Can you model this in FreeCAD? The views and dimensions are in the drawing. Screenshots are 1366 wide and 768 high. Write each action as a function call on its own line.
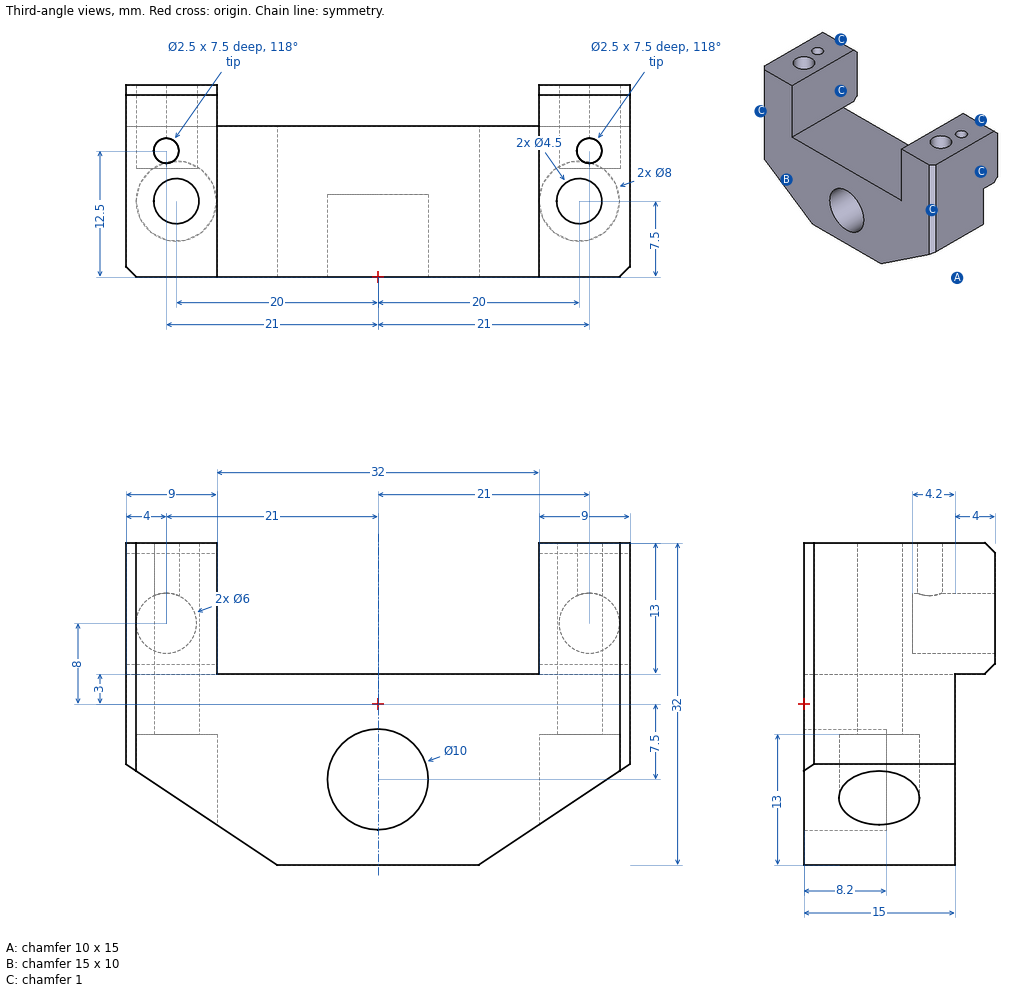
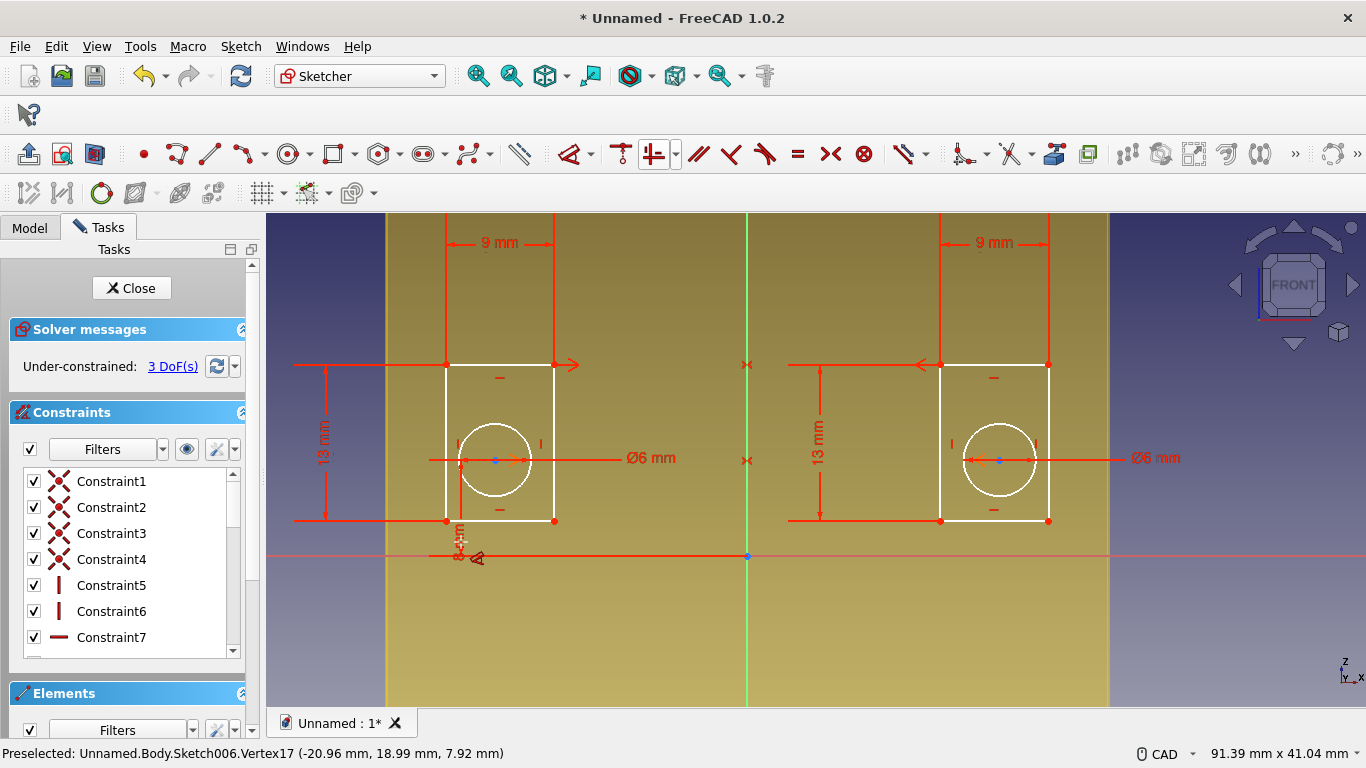
click(446, 521)
click(781, 539)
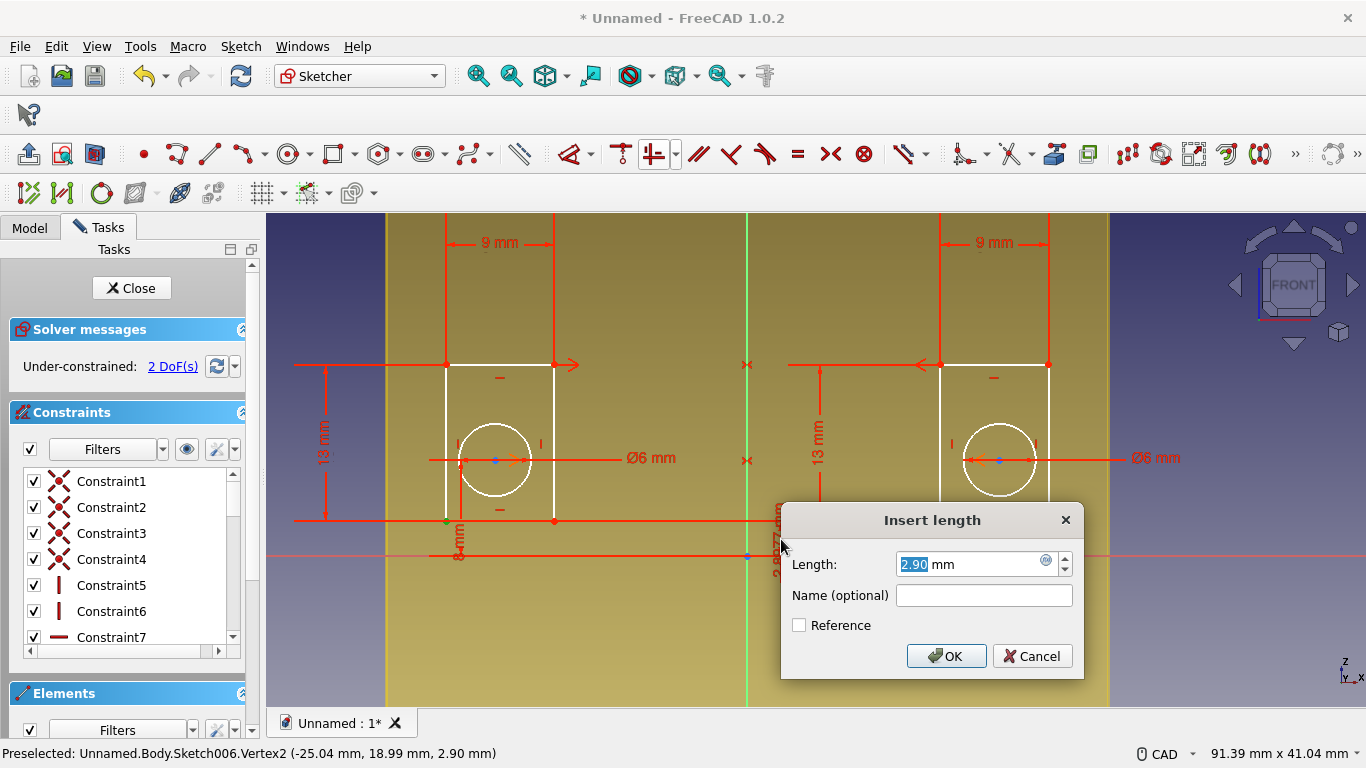
text(3)
key(Return)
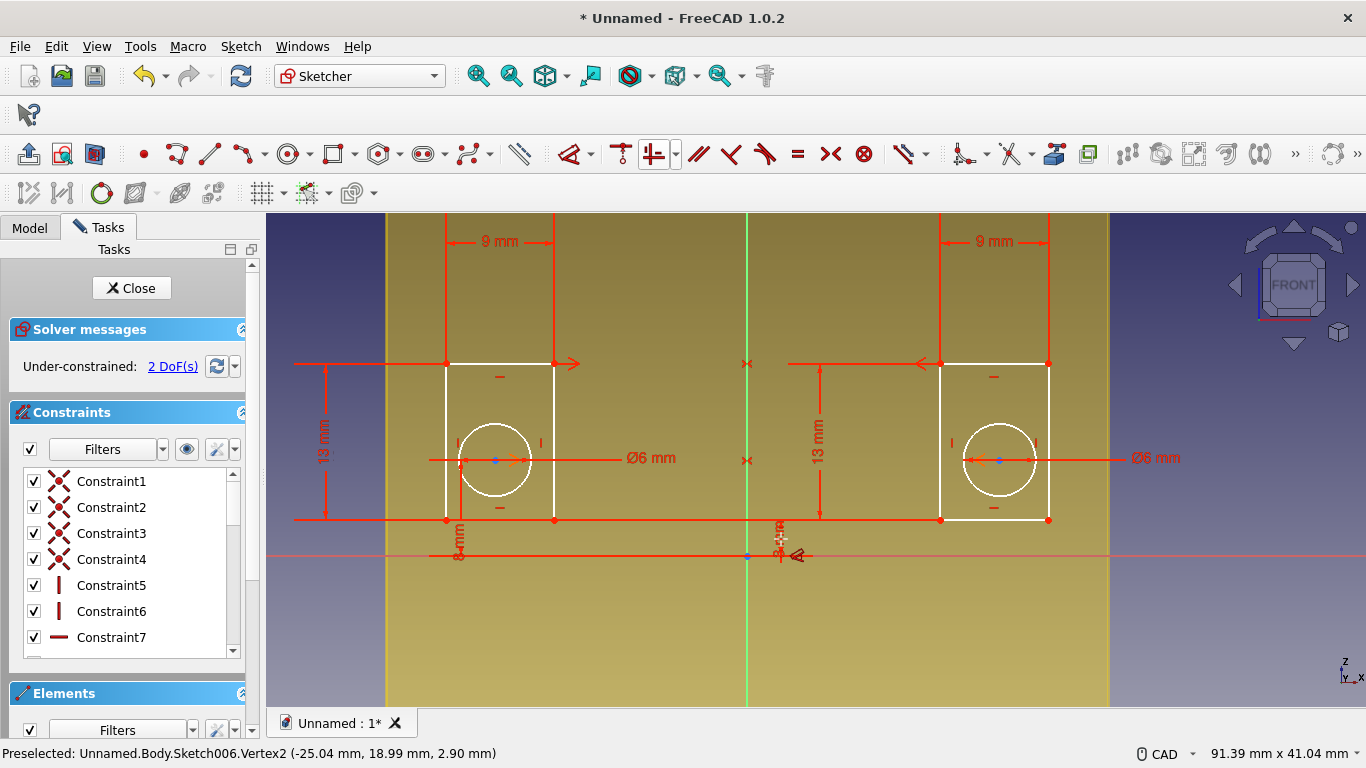
click(495, 460)
click(621, 590)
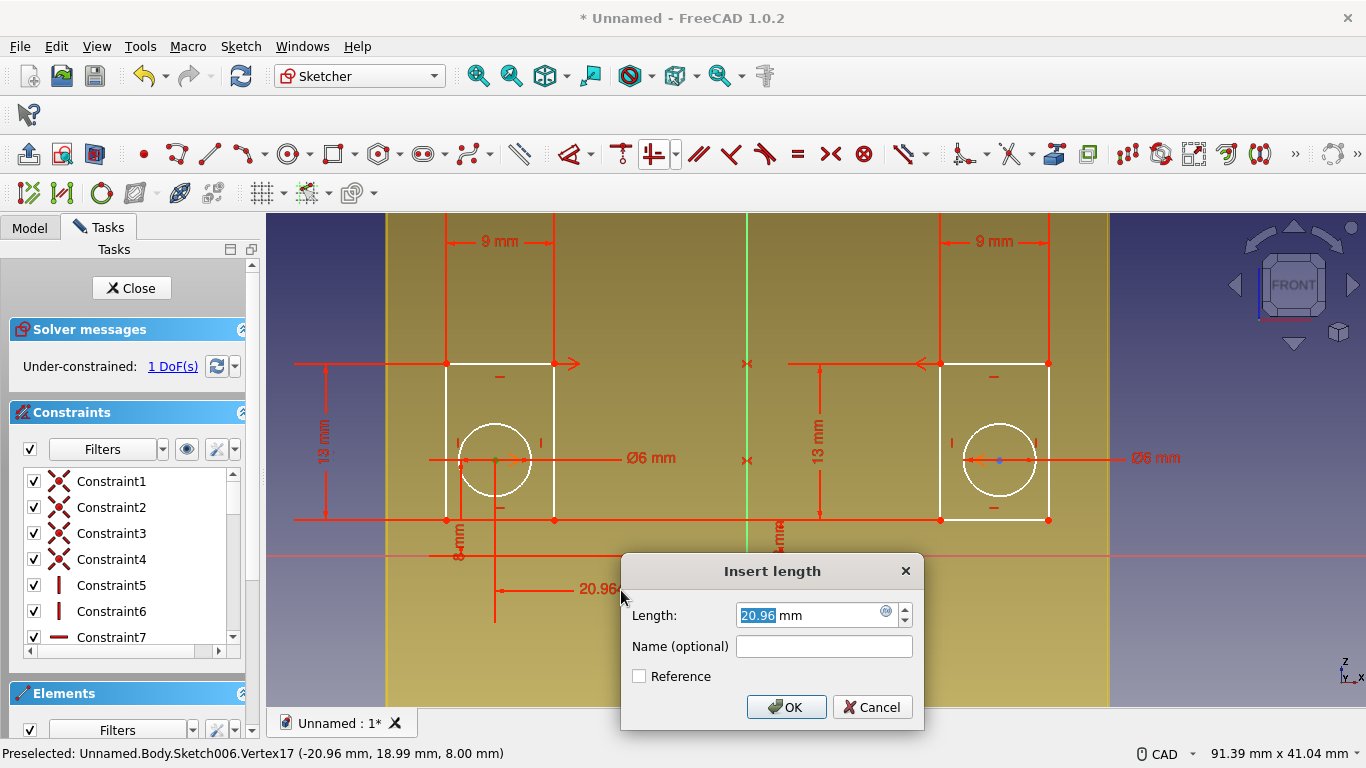
text(21)
key(Return)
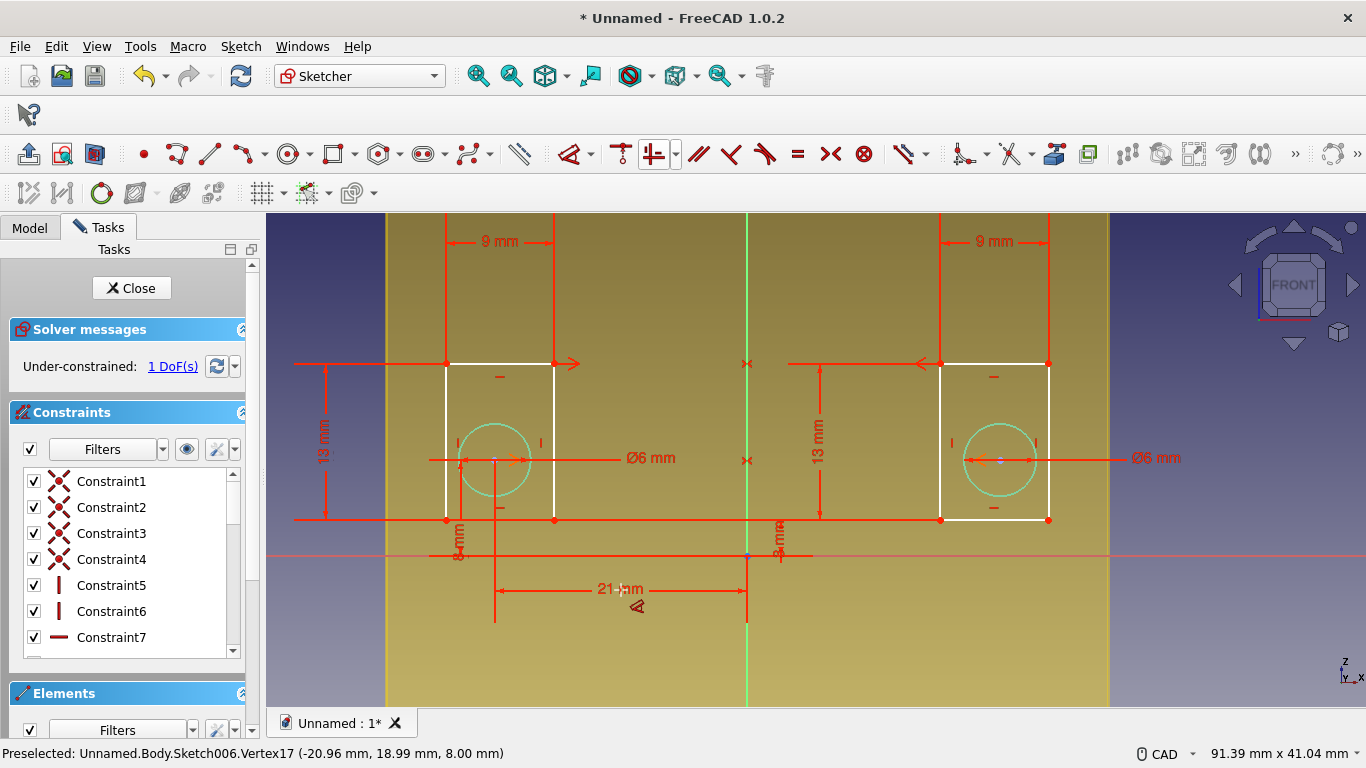
click(446, 520)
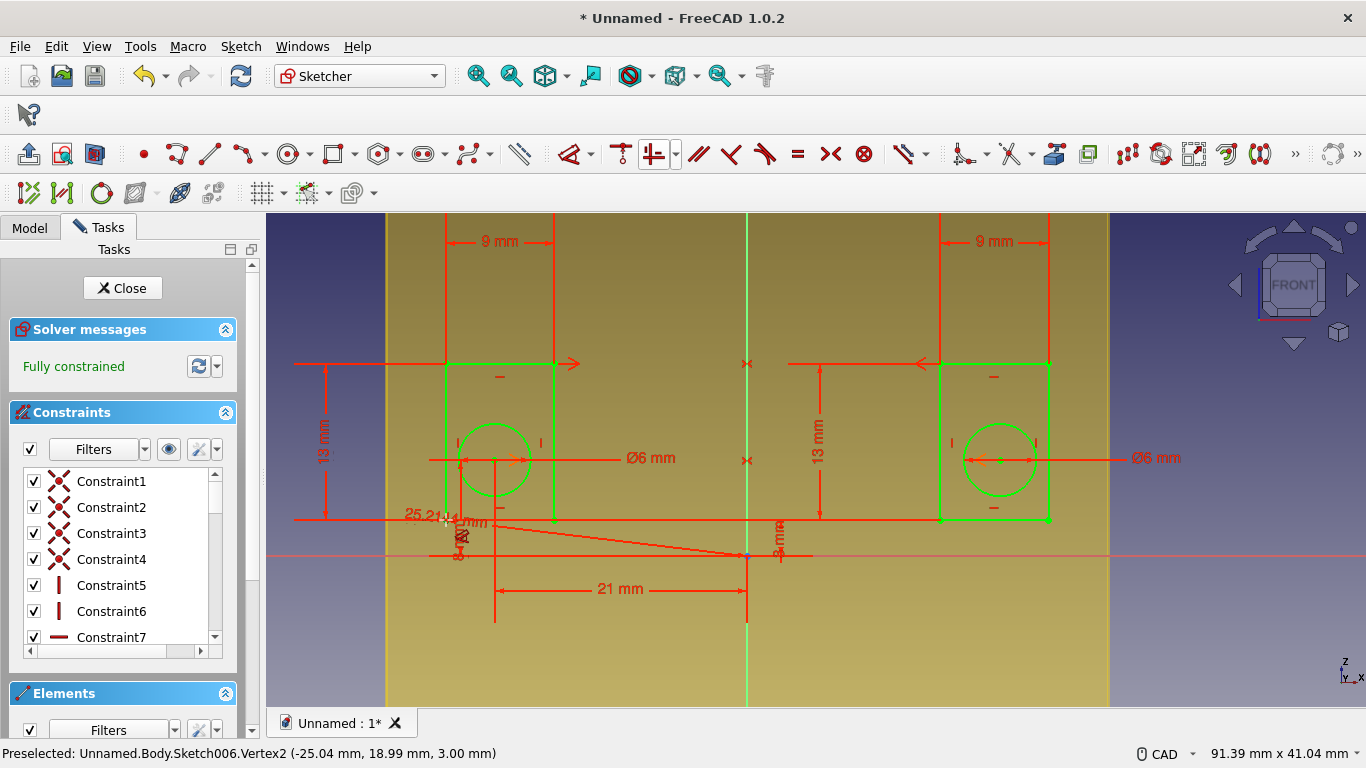
click(495, 460)
click(459, 426)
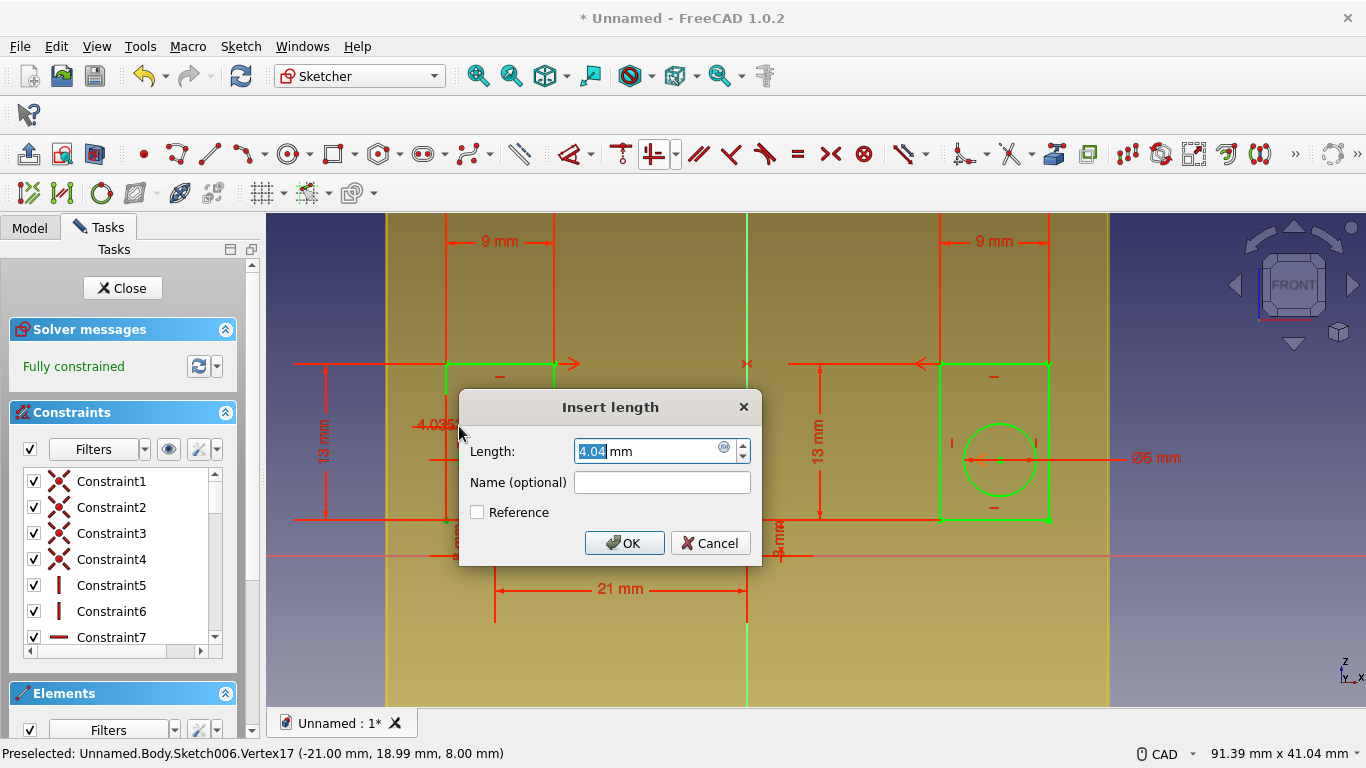
text(4)
key(Return)
key(Escape)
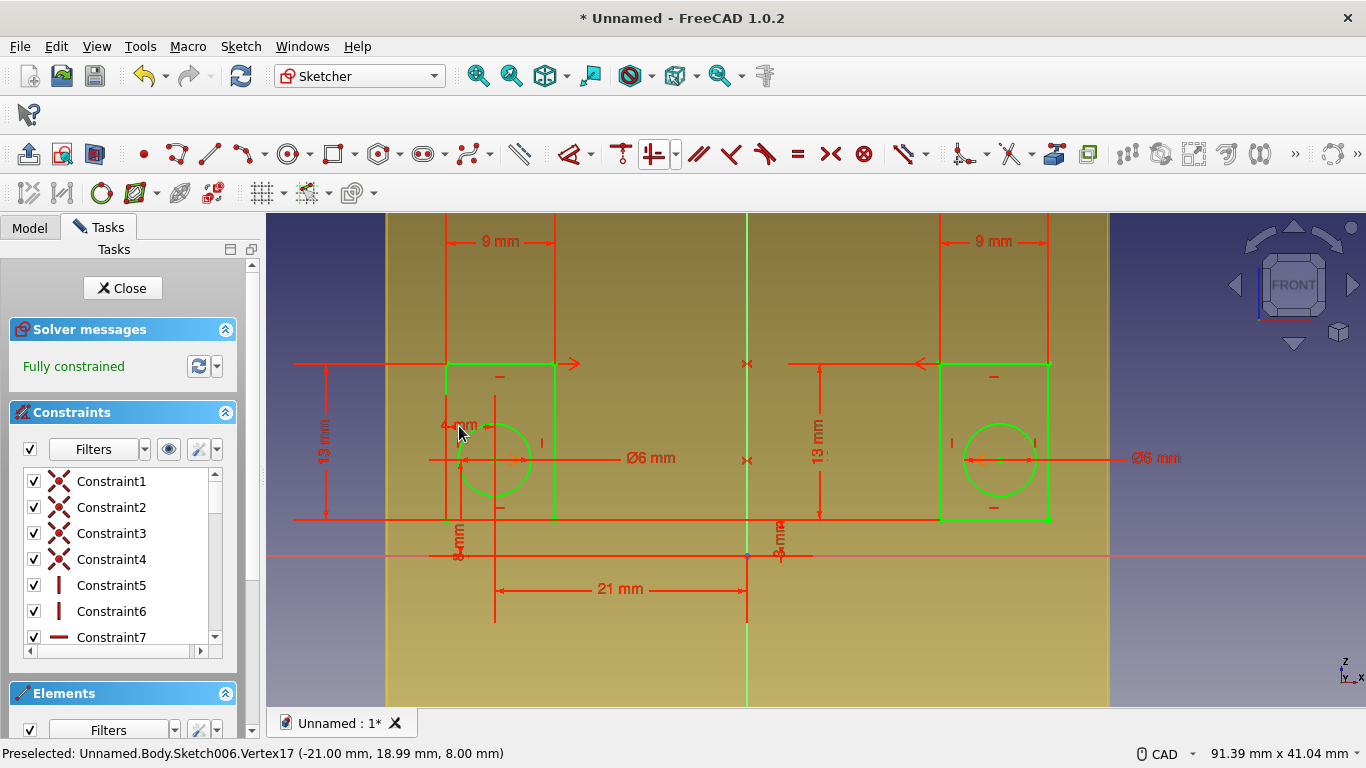
click(123, 288)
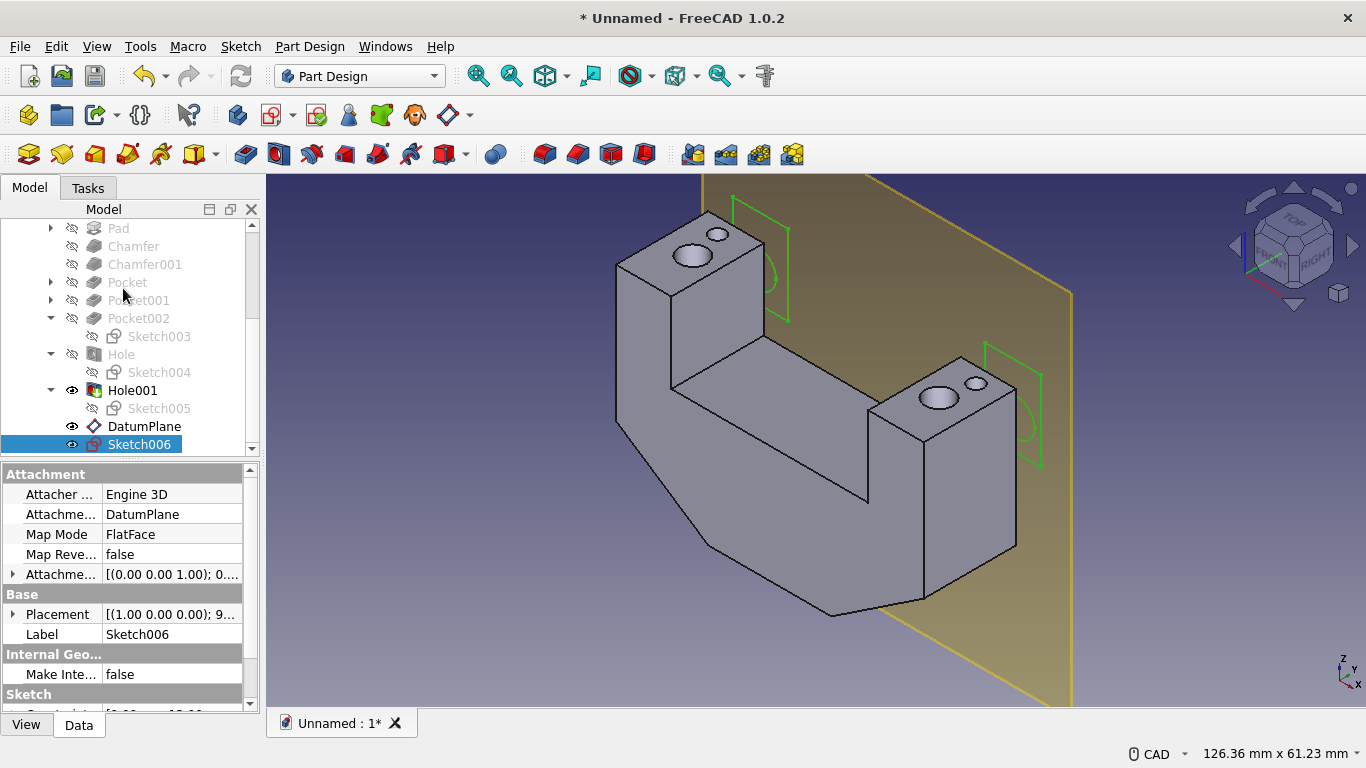
click(29, 154)